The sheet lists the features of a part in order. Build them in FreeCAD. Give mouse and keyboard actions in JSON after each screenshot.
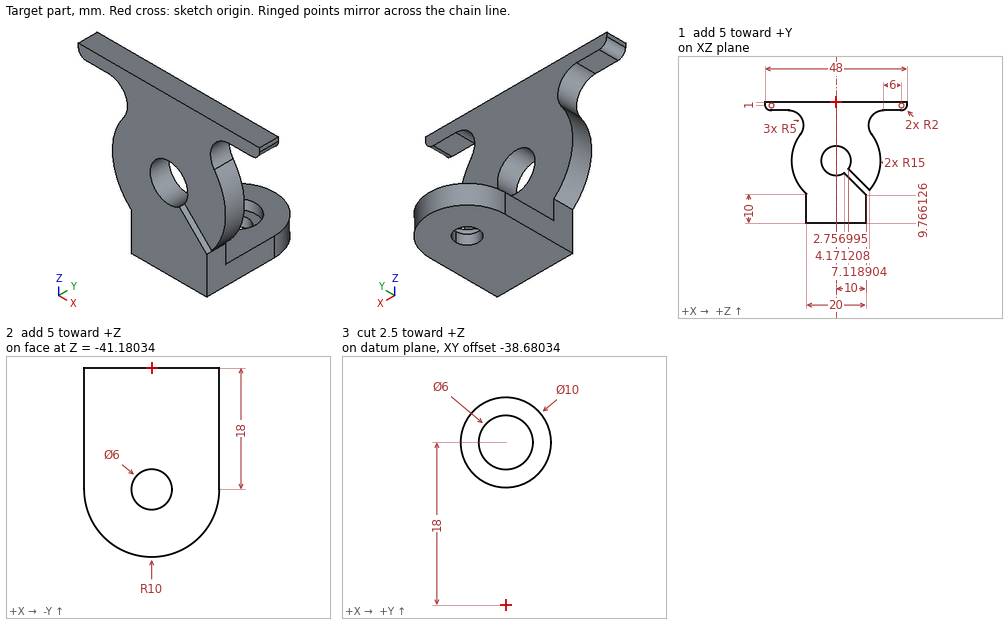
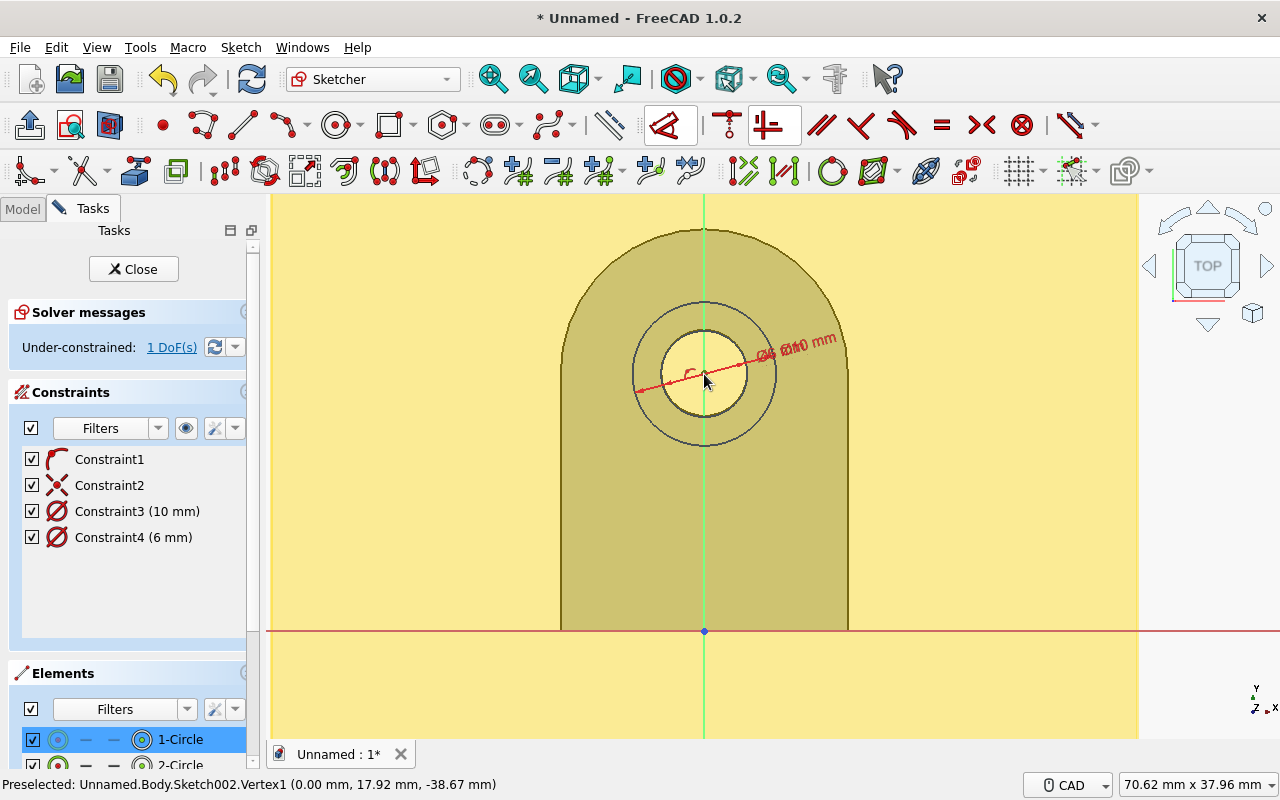
{"action": "key", "text": "i"}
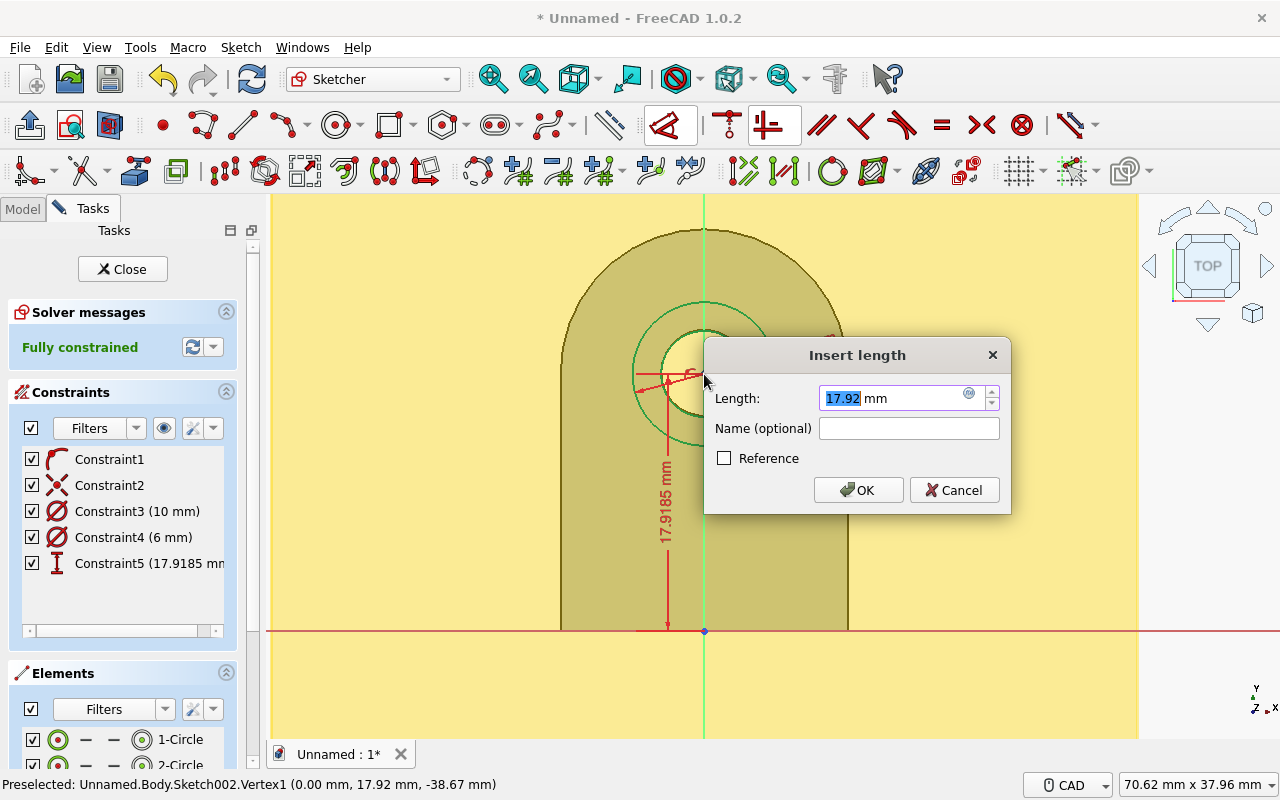
{"action": "type", "text": "18"}
{"action": "key", "text": "Return"}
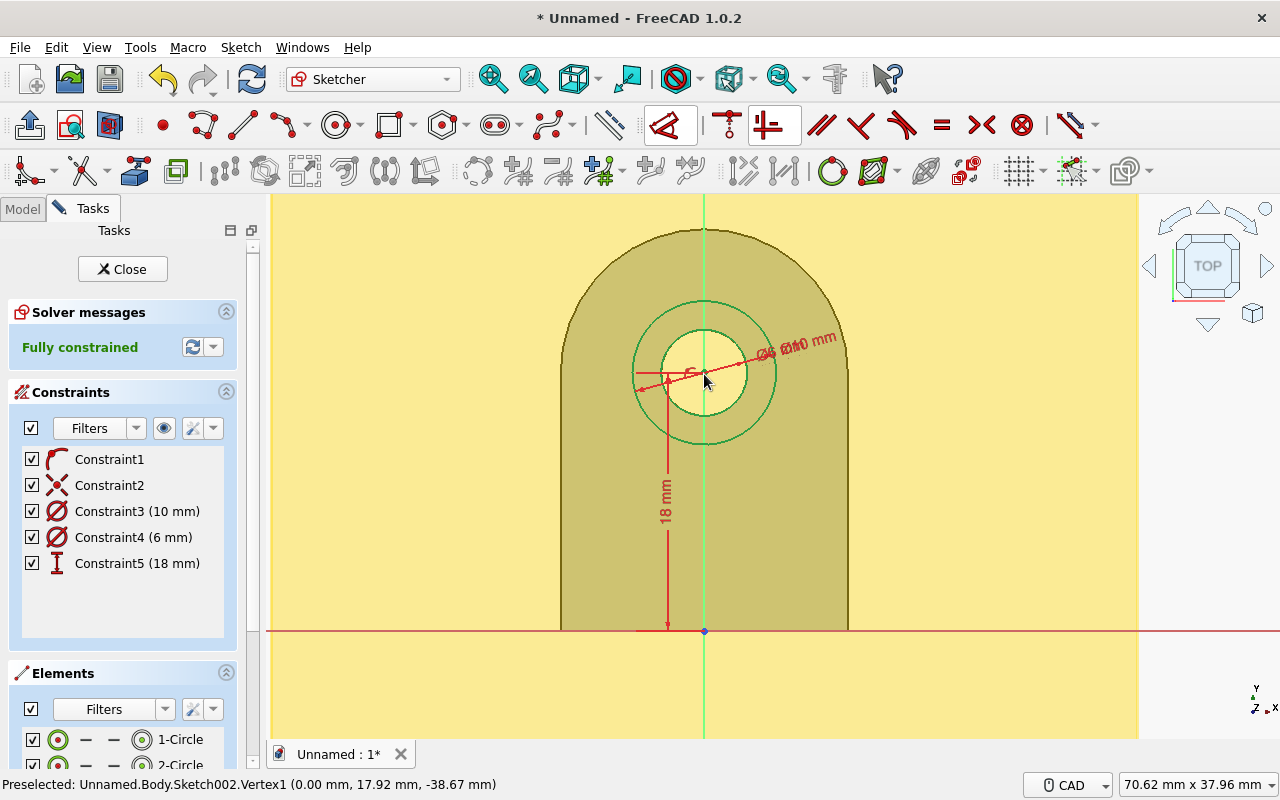
{"action": "left_click", "coordinate": [123, 269]}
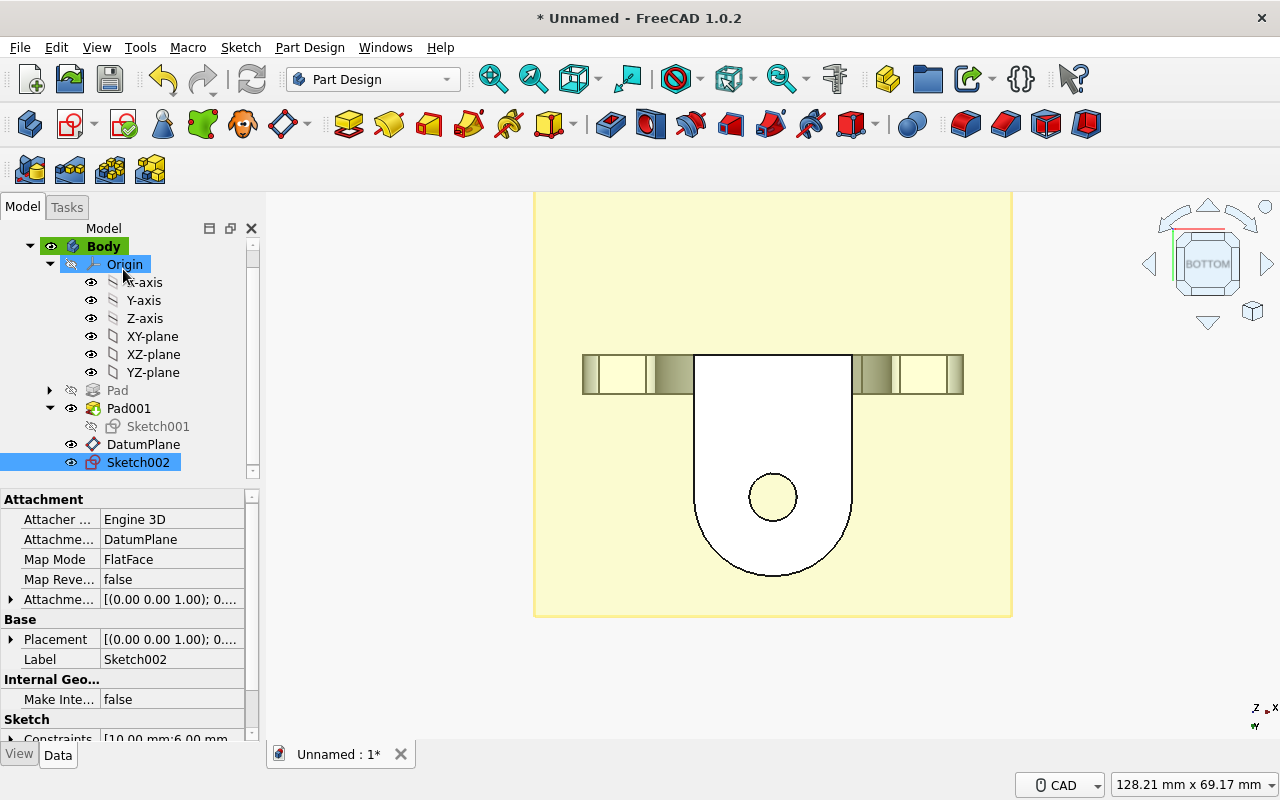
{"action": "left_click", "coordinate": [612, 124]}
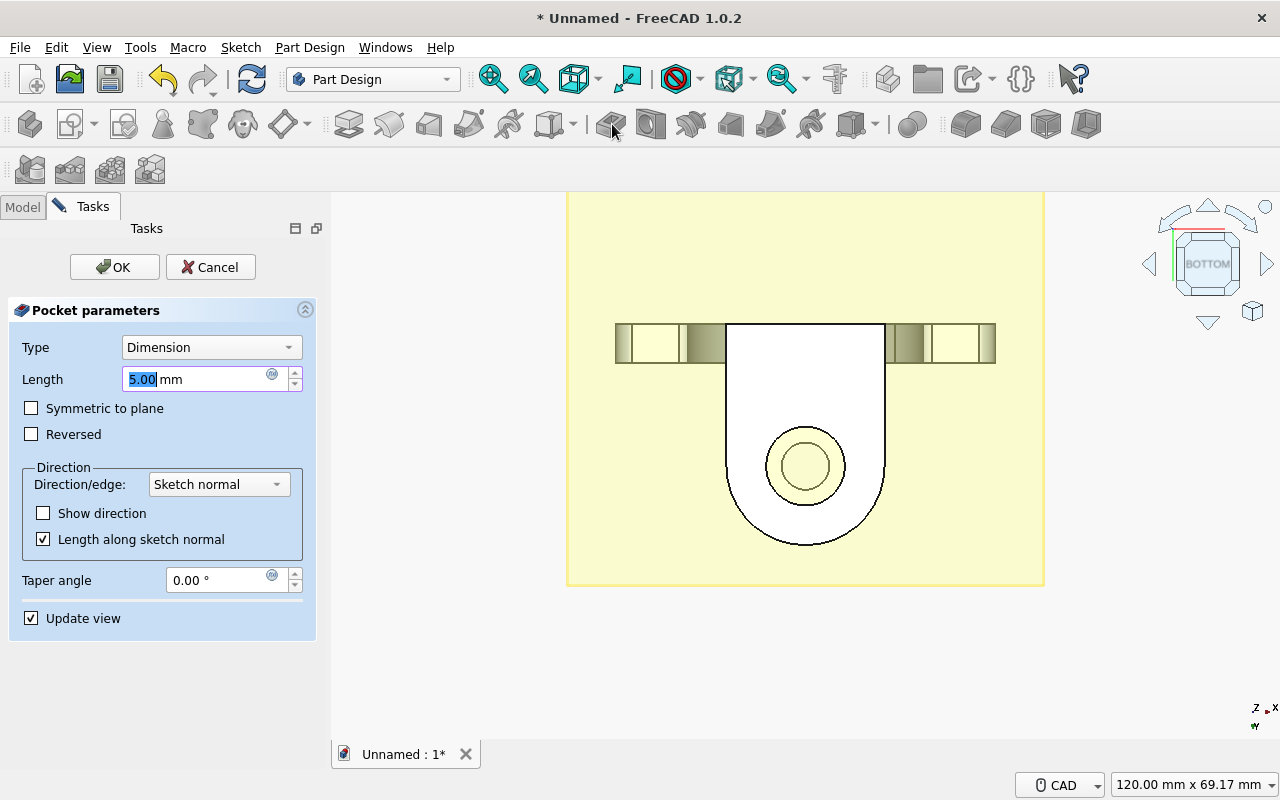
{"action": "type", "text": "2.5"}
{"action": "key", "text": "Tab"}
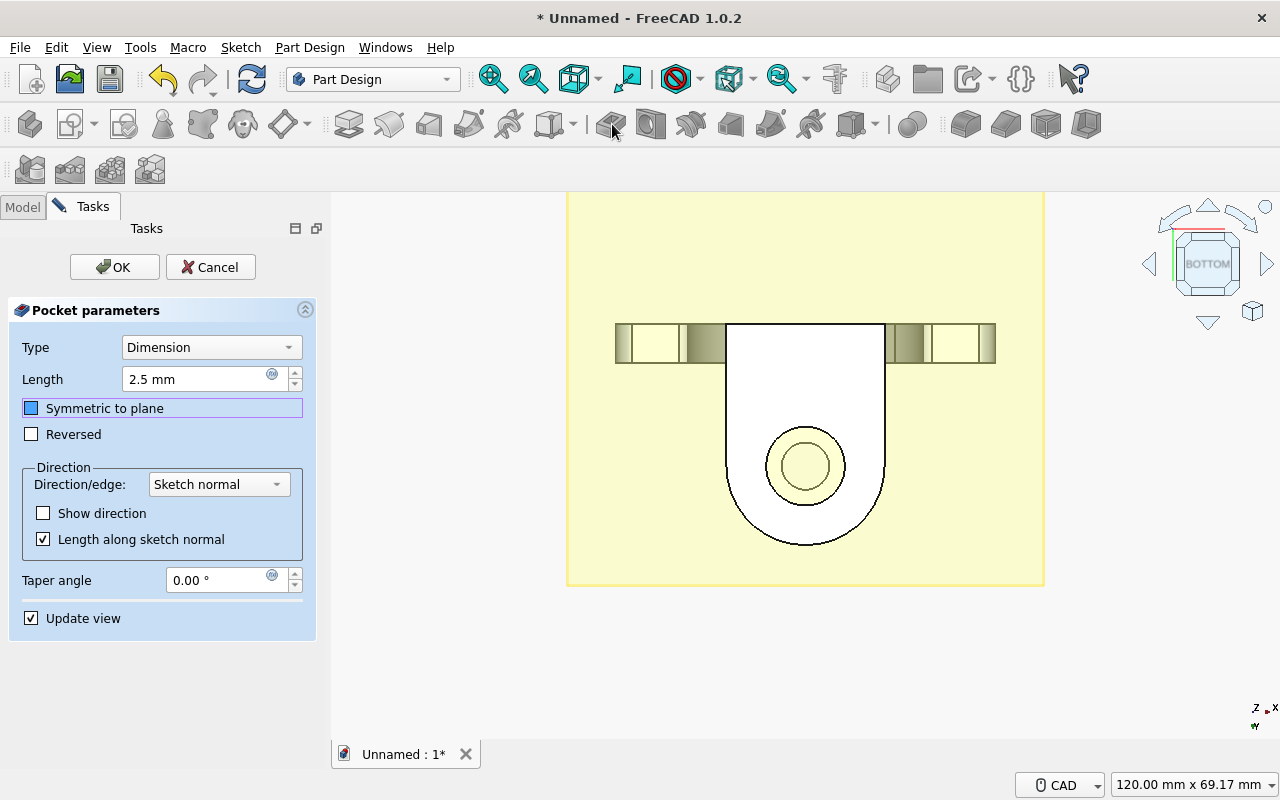
{"action": "left_click", "coordinate": [30, 434]}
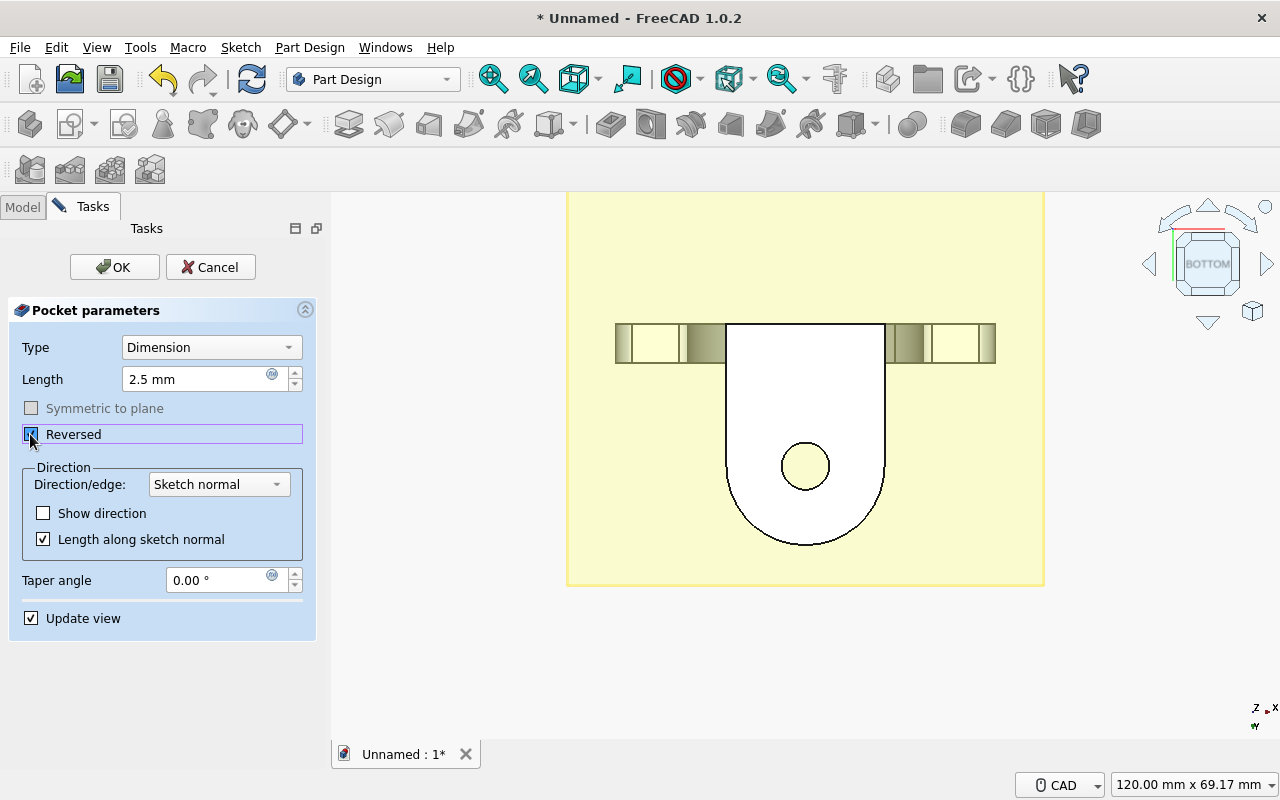
{"action": "left_click", "coordinate": [115, 267]}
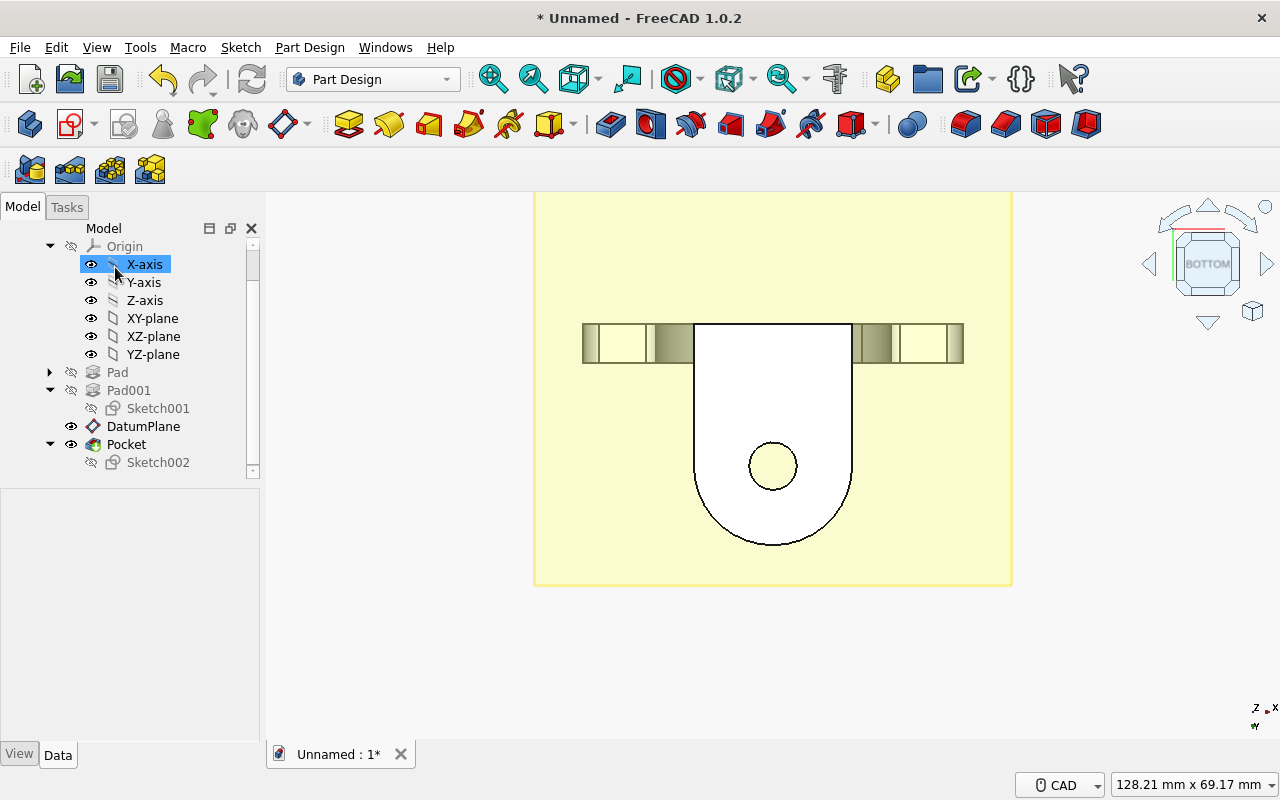
{"action": "left_click", "coordinate": [116, 426]}
{"action": "key", "text": "space"}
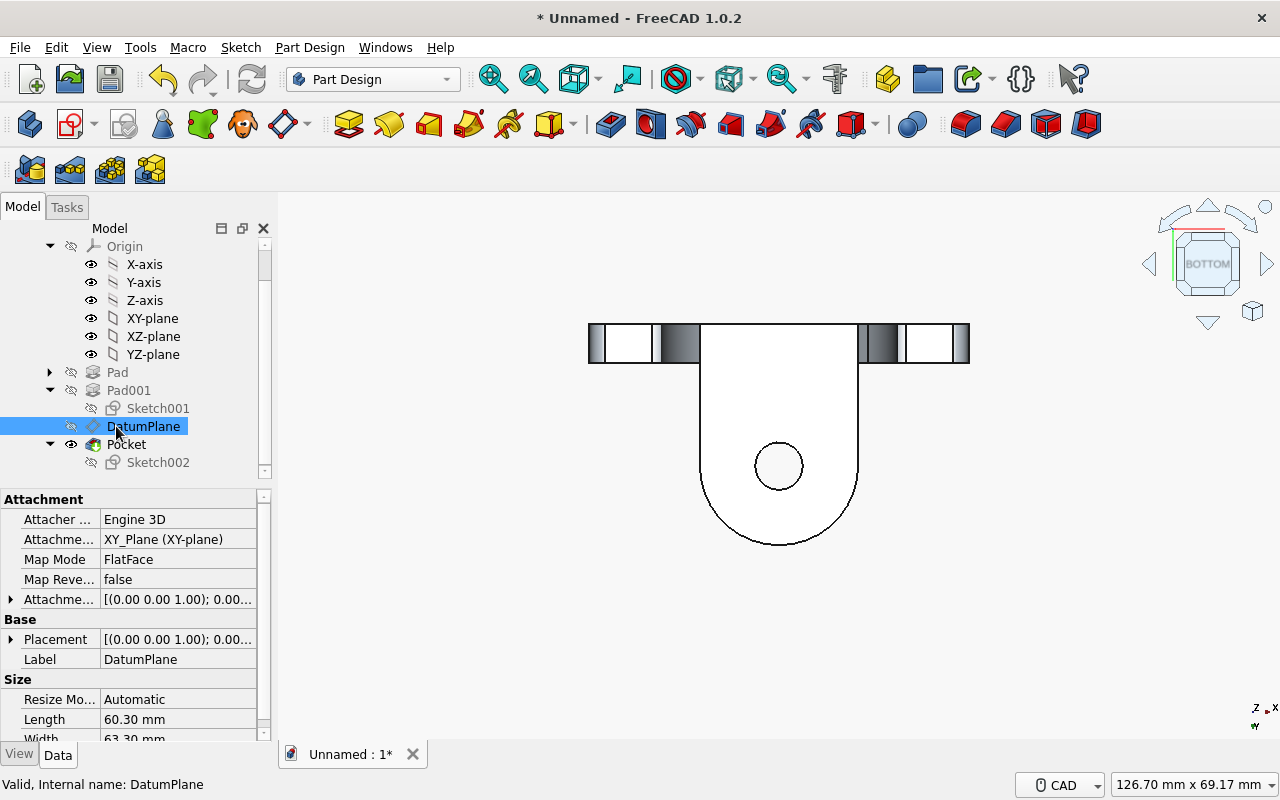
{"action": "key", "text": "0"}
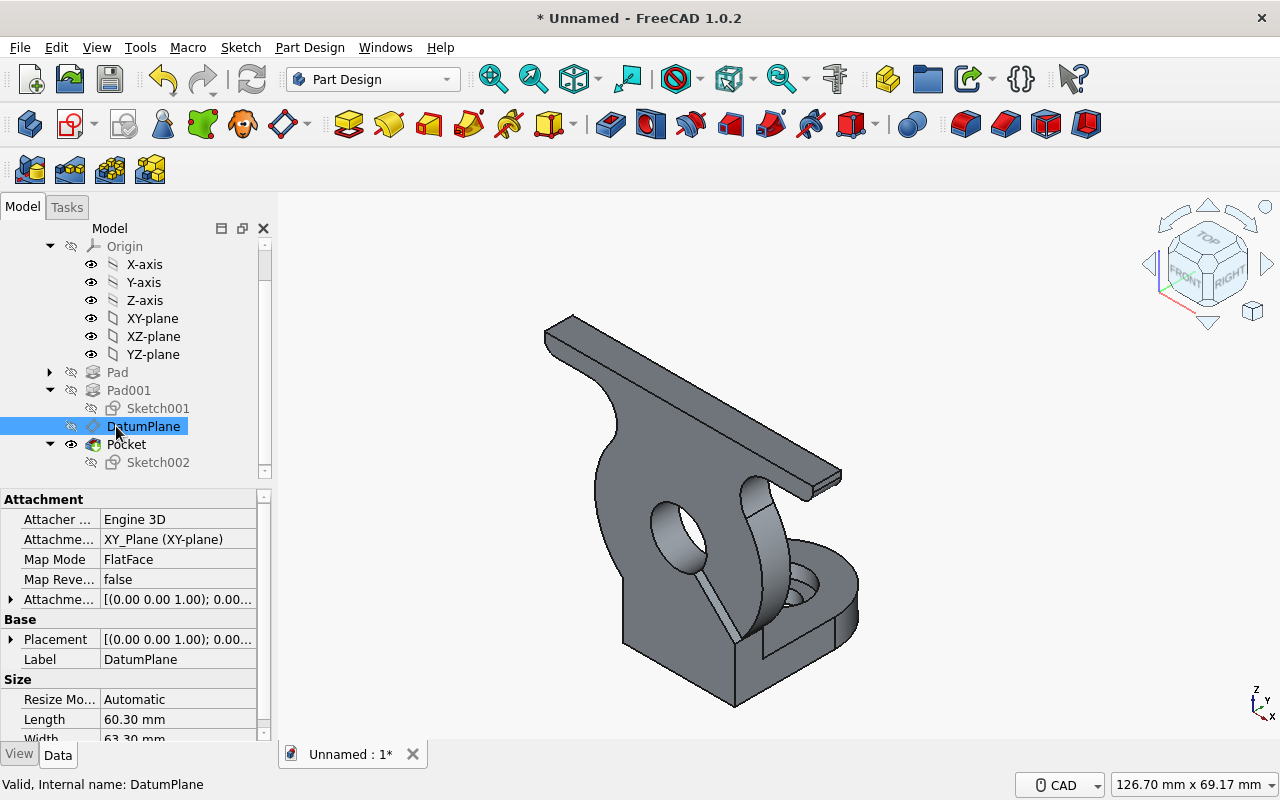
{"action": "key", "text": "v f"}